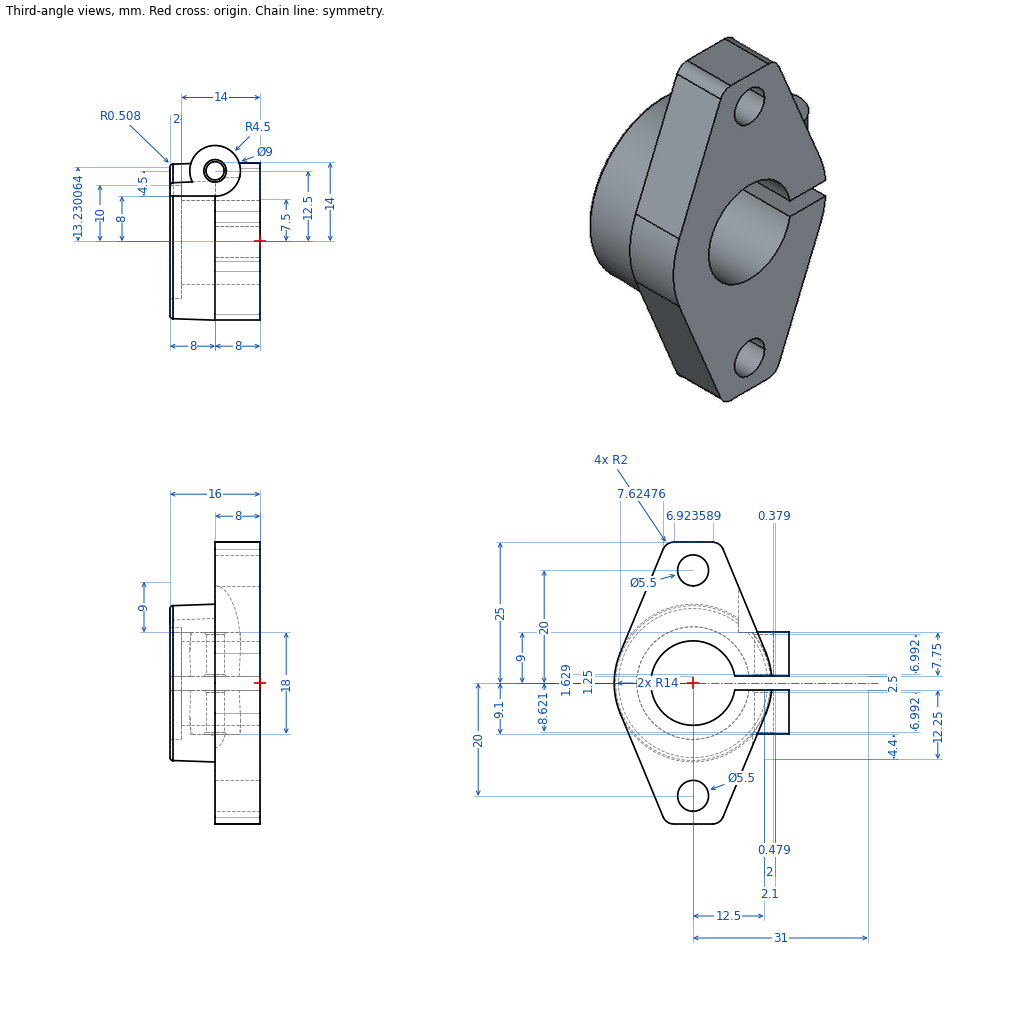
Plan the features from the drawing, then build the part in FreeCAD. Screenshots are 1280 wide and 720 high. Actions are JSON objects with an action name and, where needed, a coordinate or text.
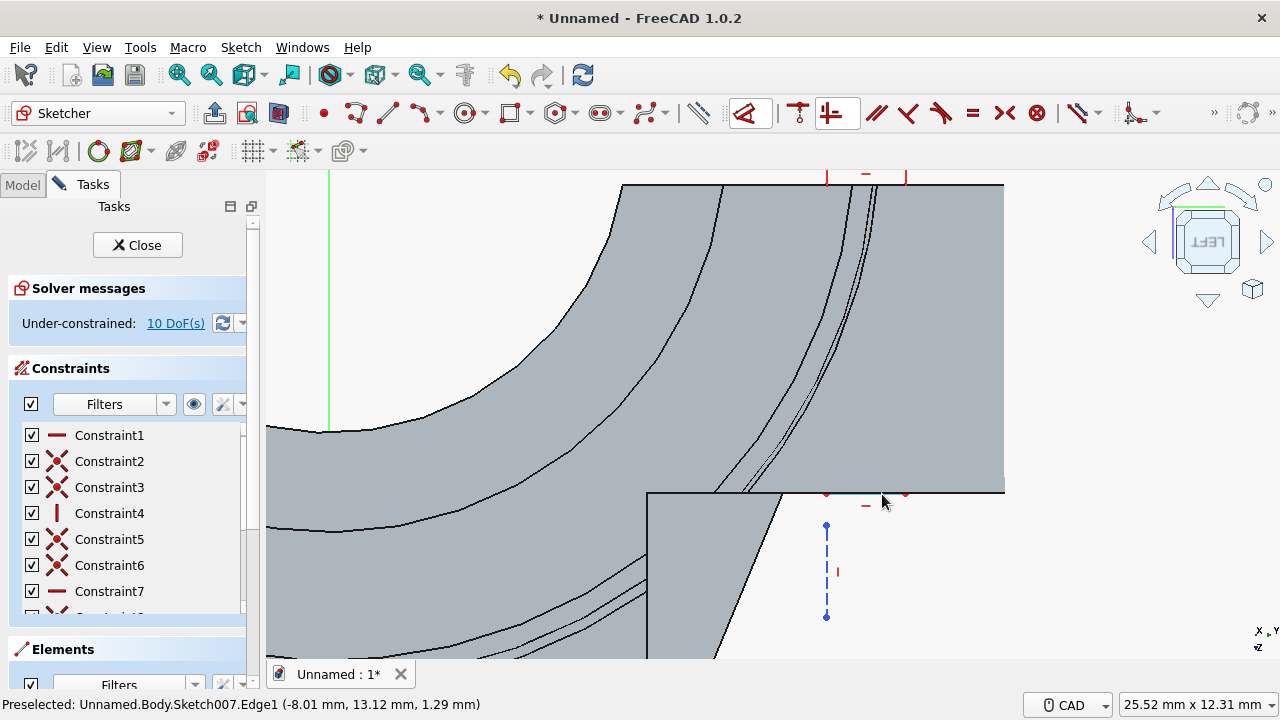
{"action": "left_click", "coordinate": [882, 494]}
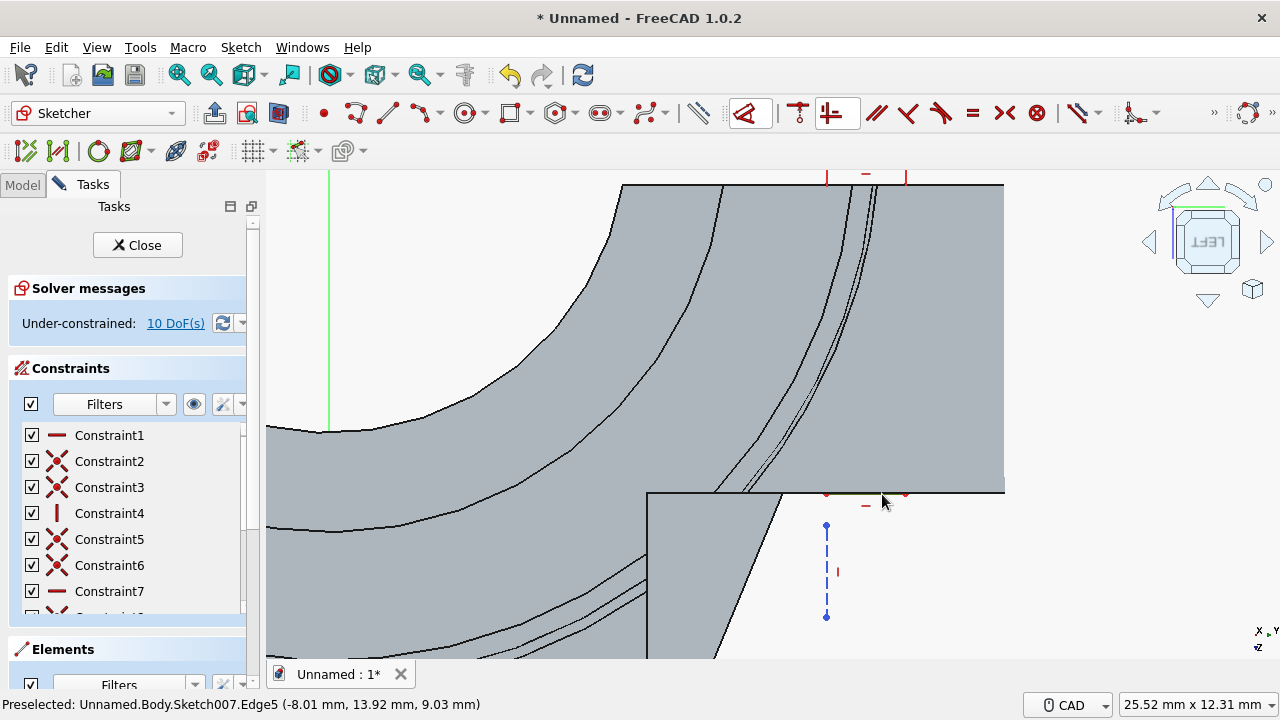
{"action": "left_click", "coordinate": [766, 114]}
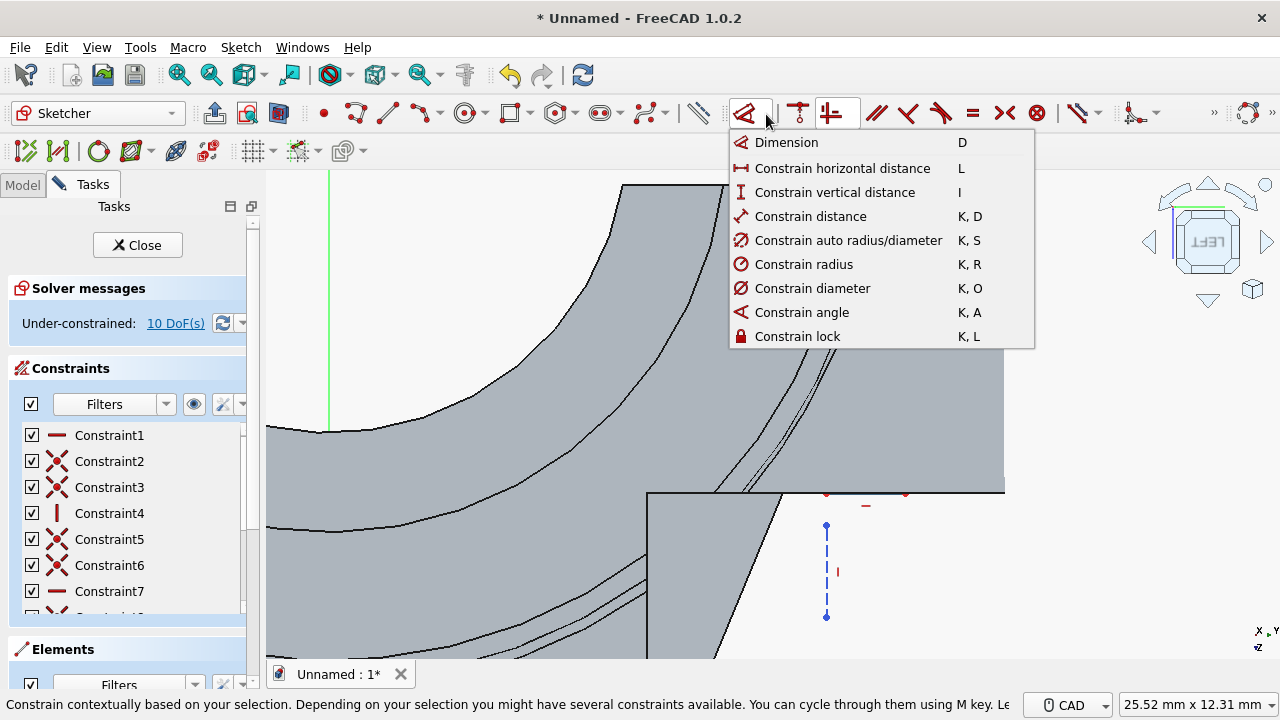
{"action": "left_click", "coordinate": [882, 168]}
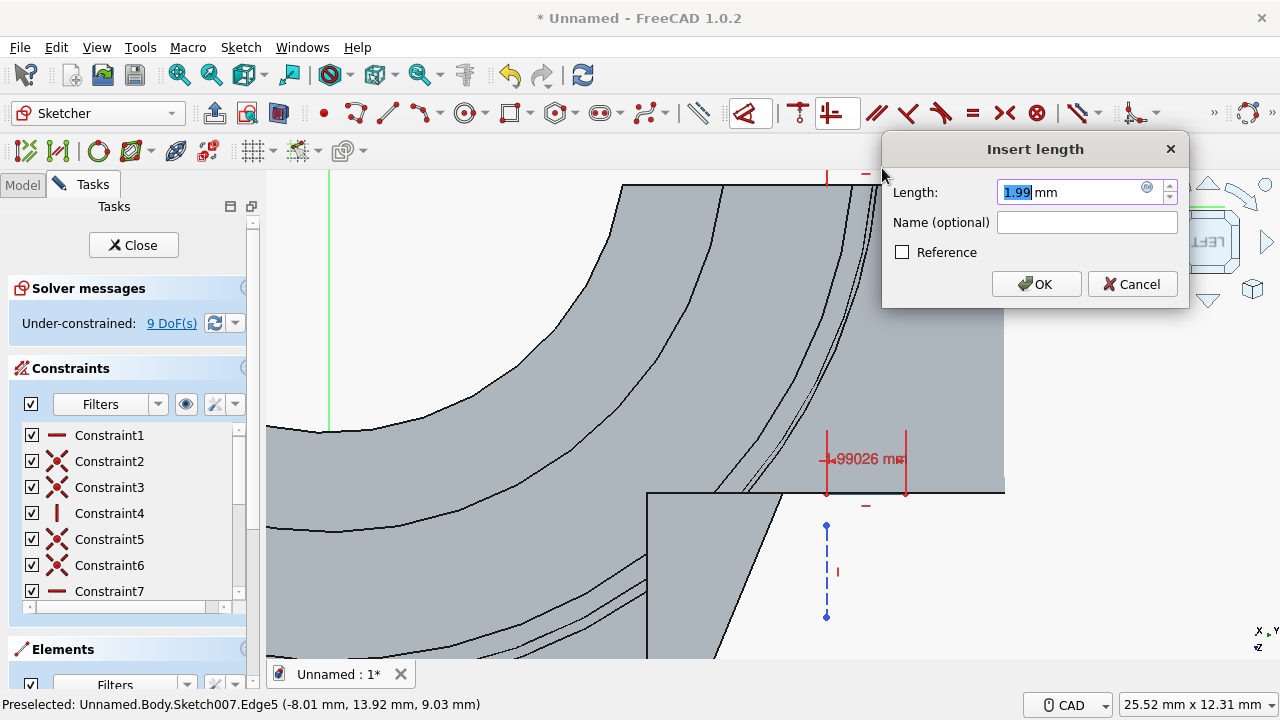
{"action": "type", "text": "2"}
{"action": "key", "text": "Return"}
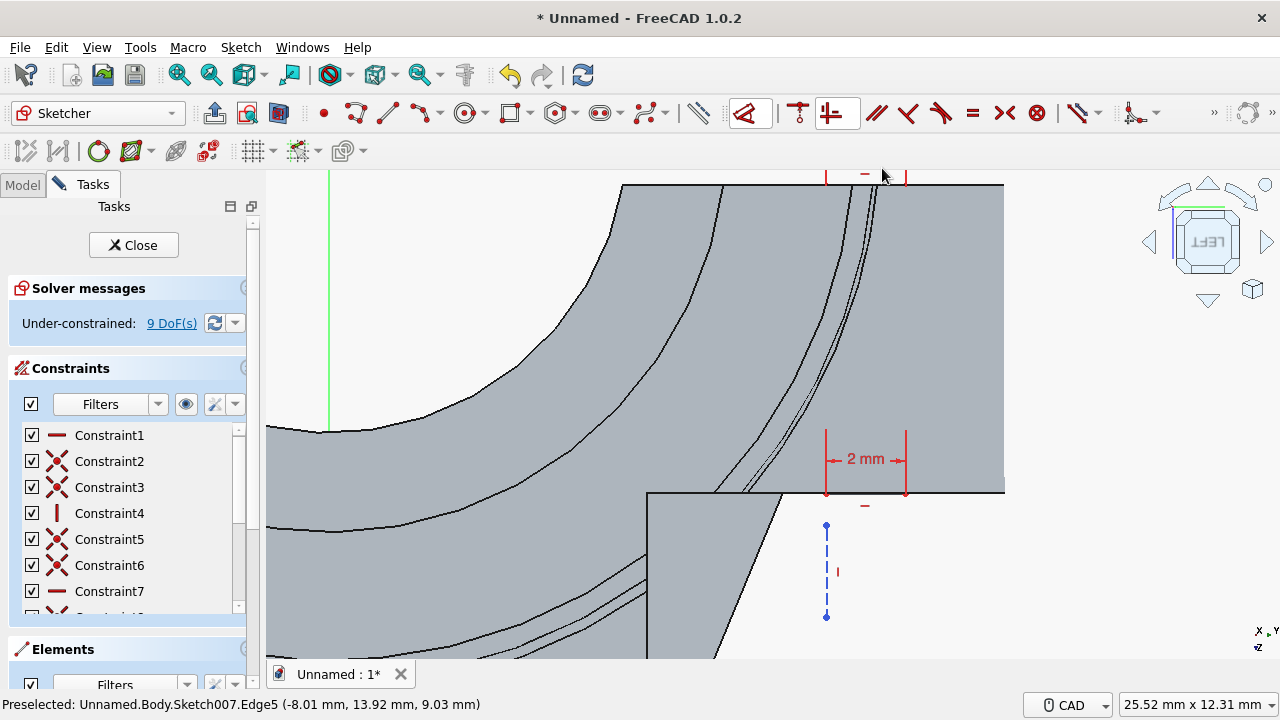
{"action": "left_click", "coordinate": [906, 494]}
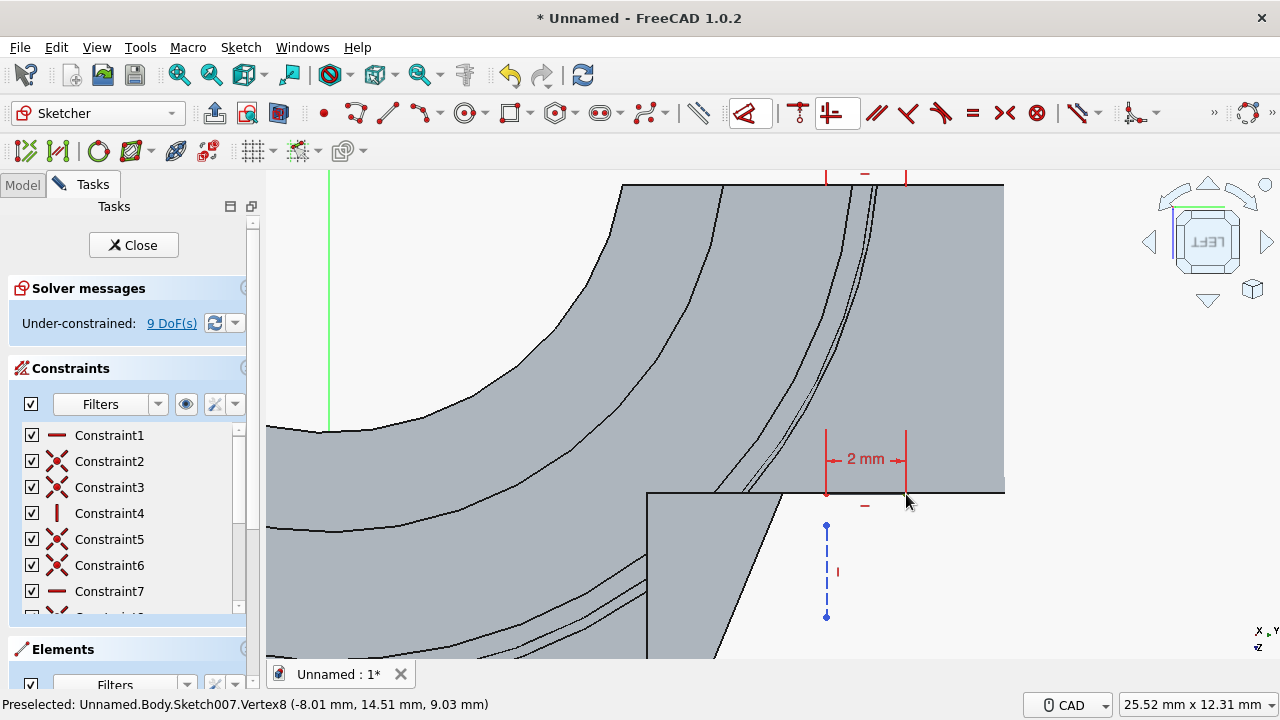
{"action": "left_click", "coordinate": [766, 114]}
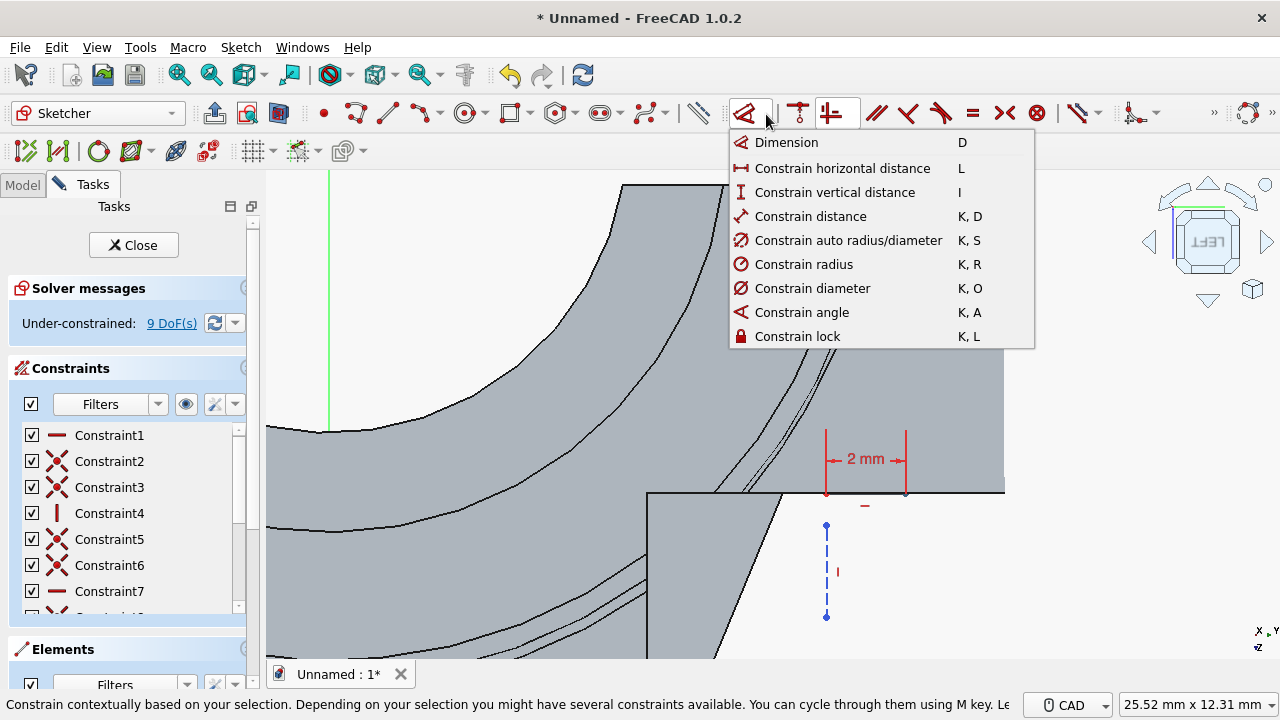
{"action": "left_click", "coordinate": [882, 192]}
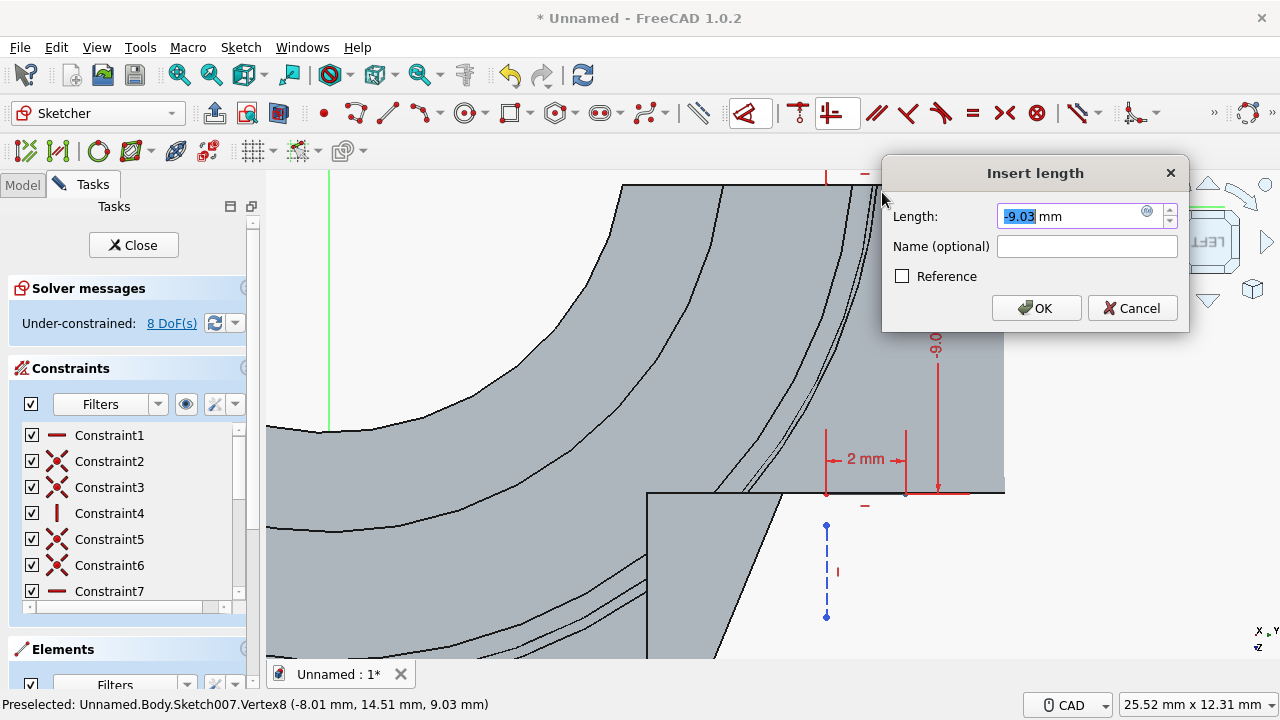
{"action": "type", "text": "-9"}
{"action": "key", "text": "Return"}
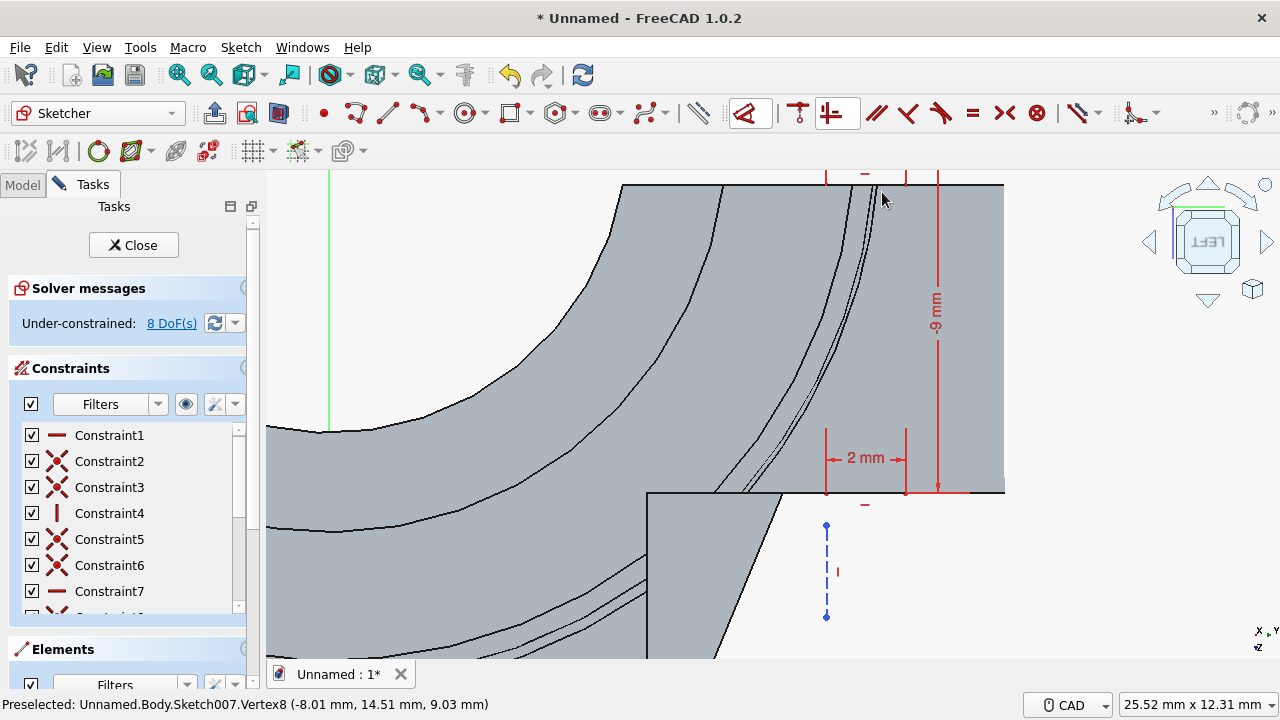
{"action": "left_click", "coordinate": [826, 401]}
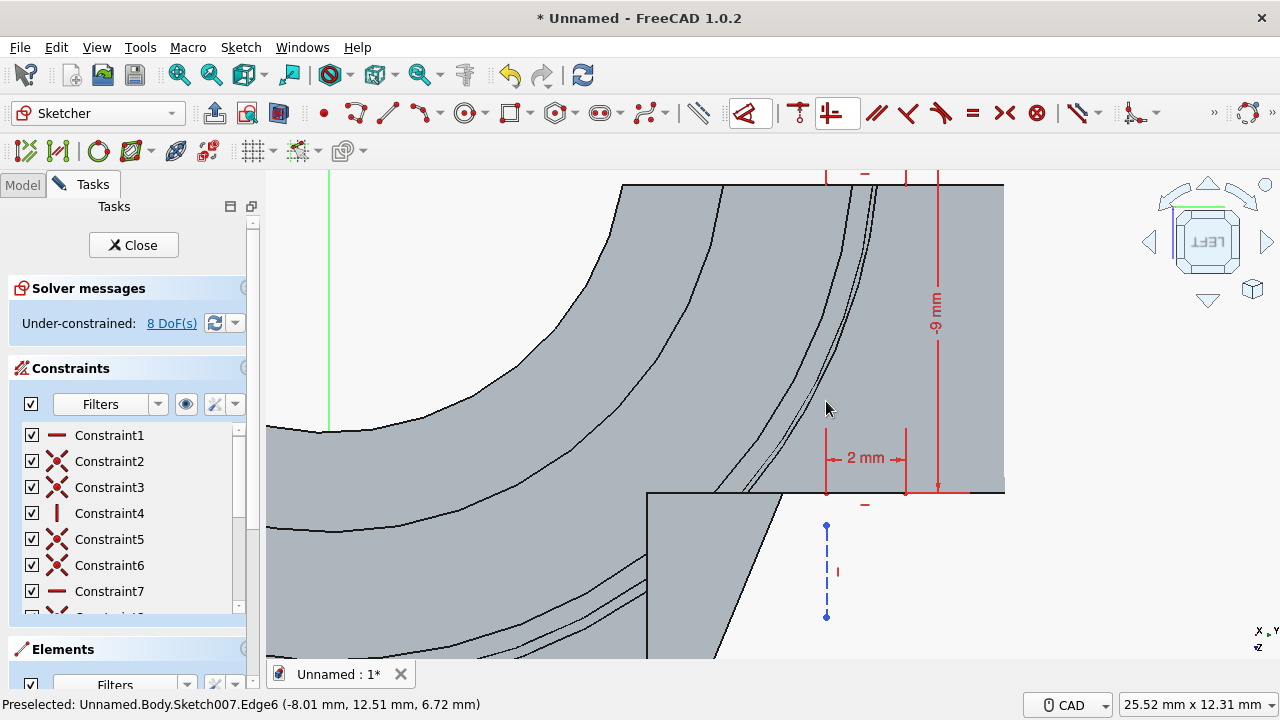
{"action": "key", "text": "i"}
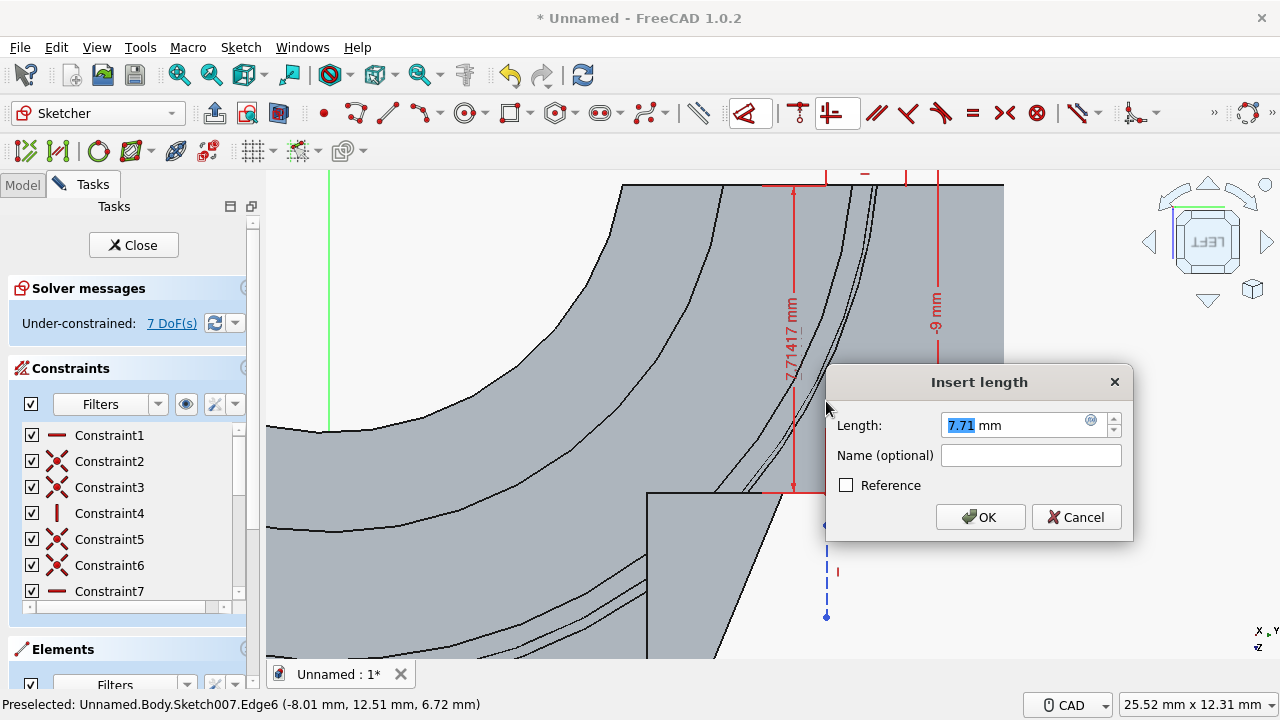
{"action": "type", "text": "7.75"}
{"action": "key", "text": "Return"}